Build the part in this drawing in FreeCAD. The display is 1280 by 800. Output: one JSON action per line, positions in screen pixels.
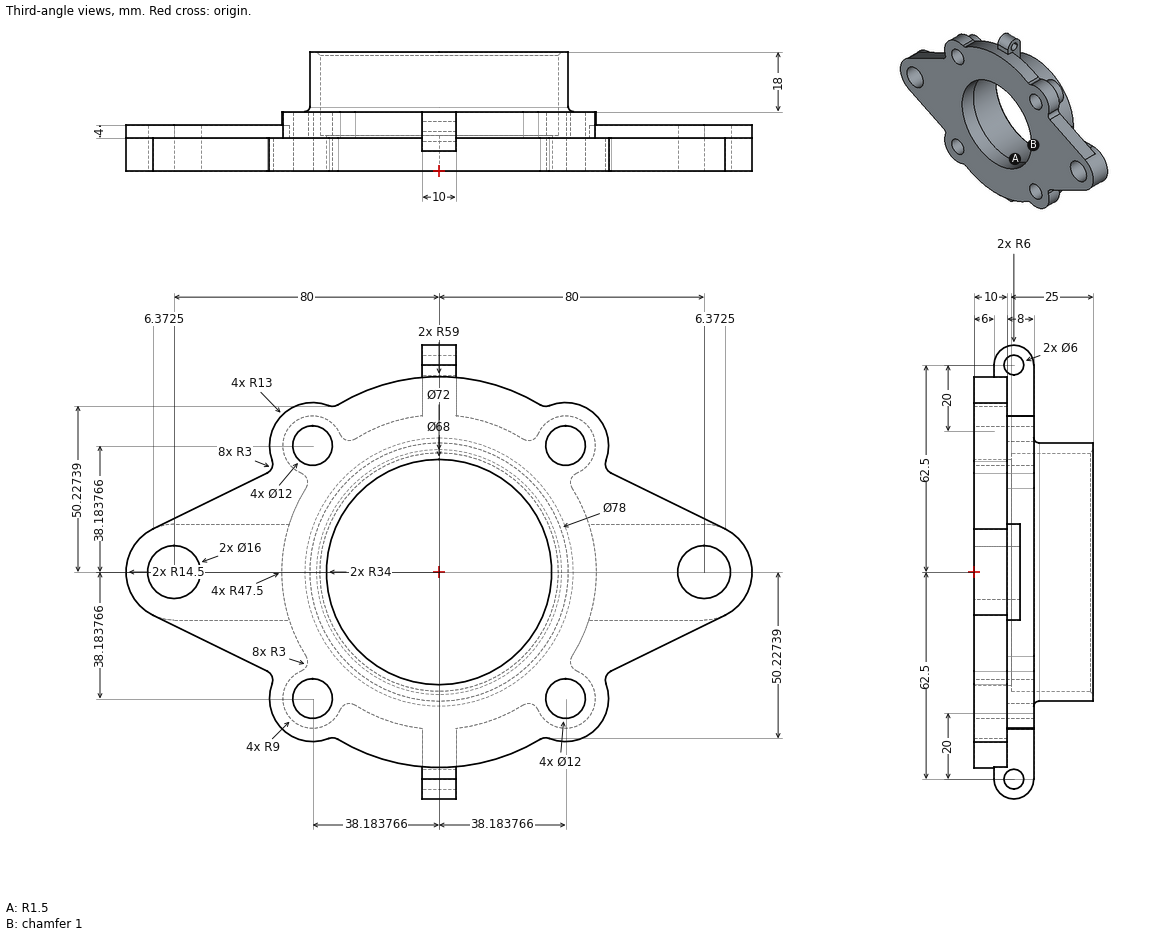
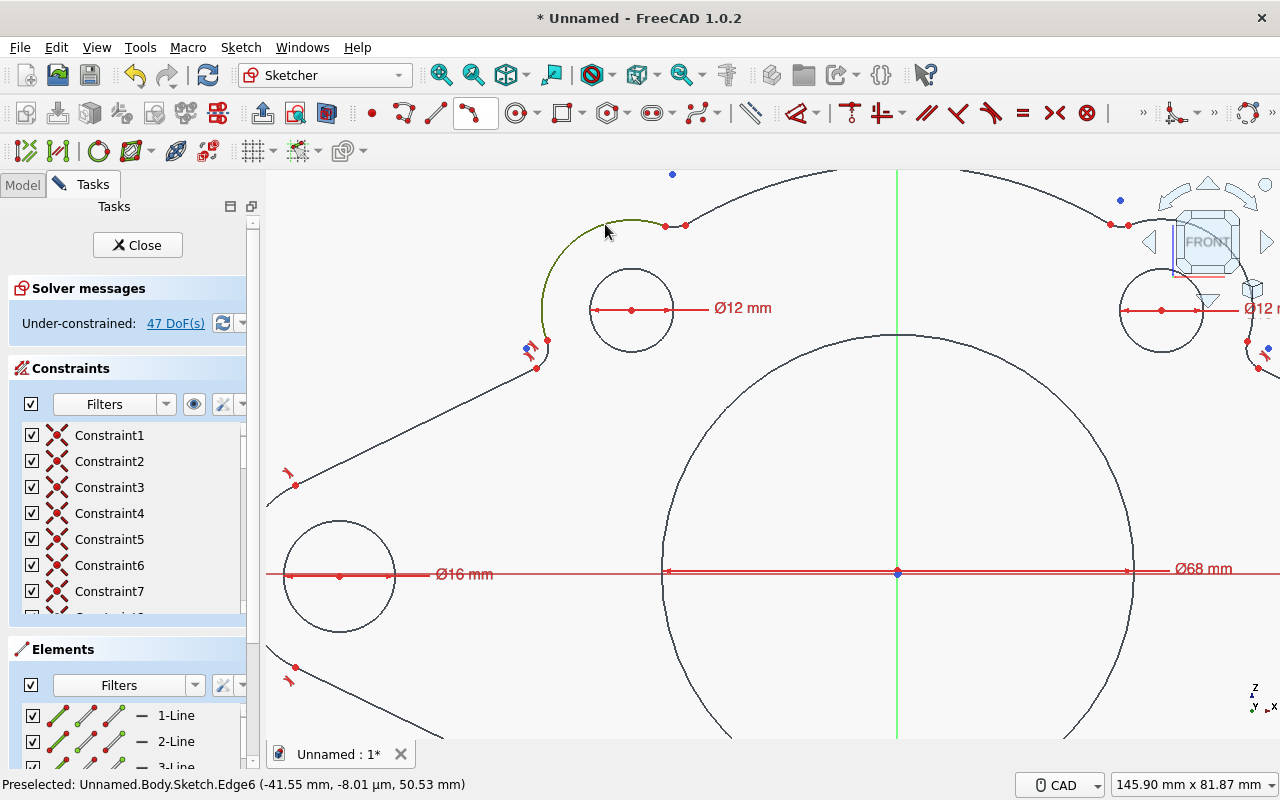
{"action": "scroll", "coordinate": [675, 227], "scroll_direction": "up", "scroll_amount": 2}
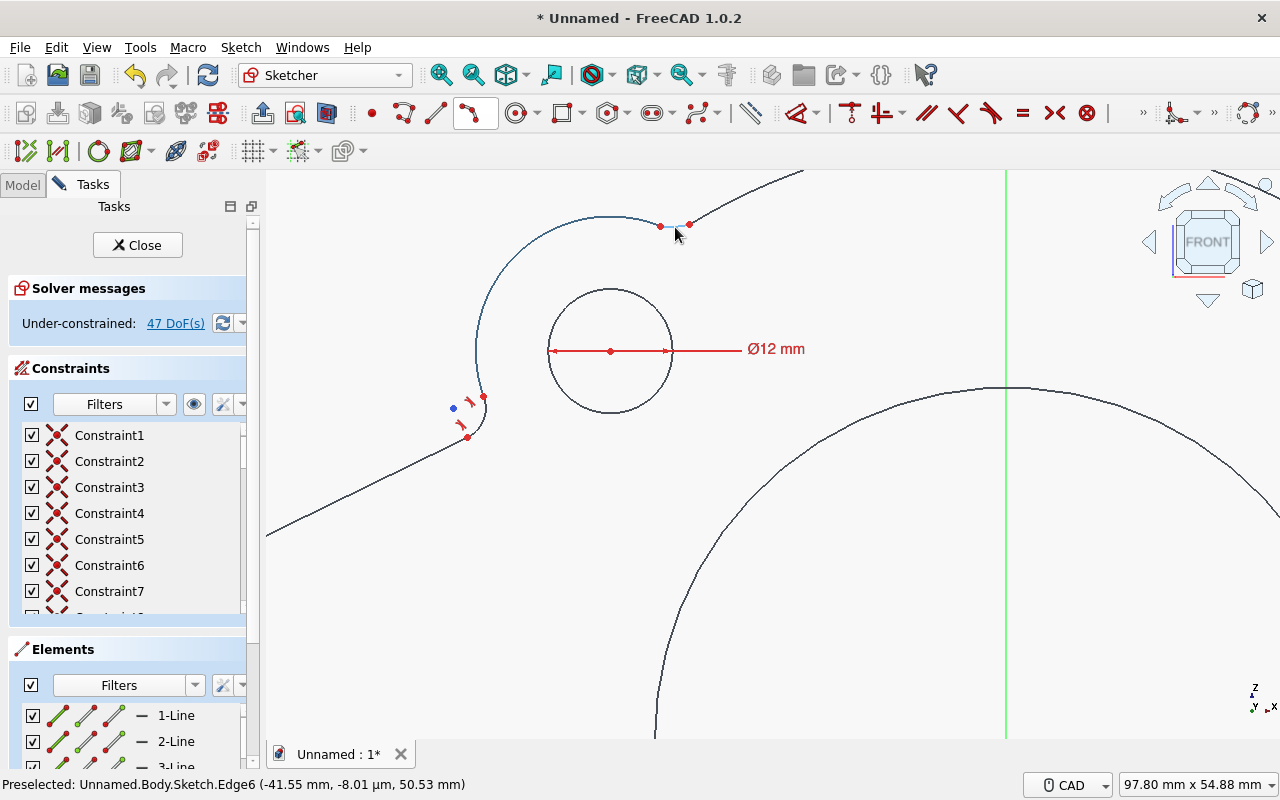
{"action": "left_click", "coordinate": [675, 227]}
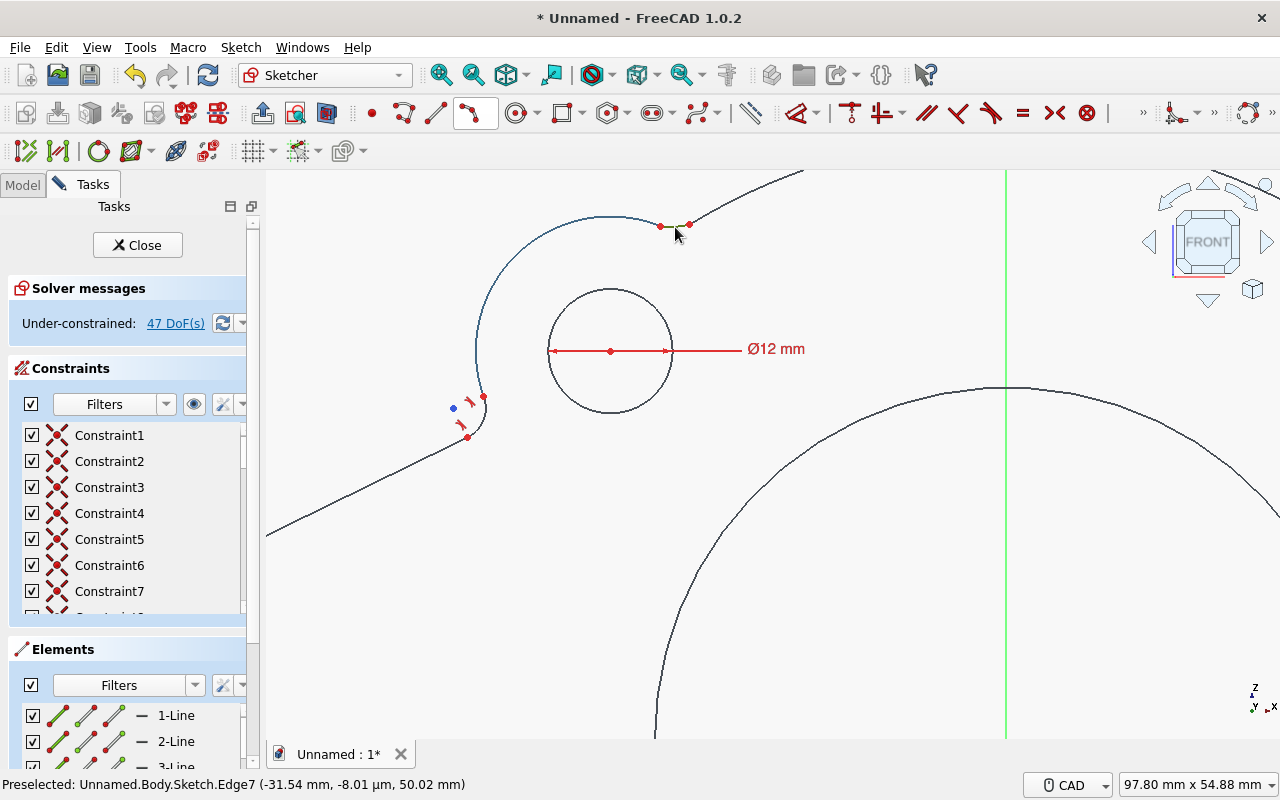
{"action": "left_click", "coordinate": [992, 114]}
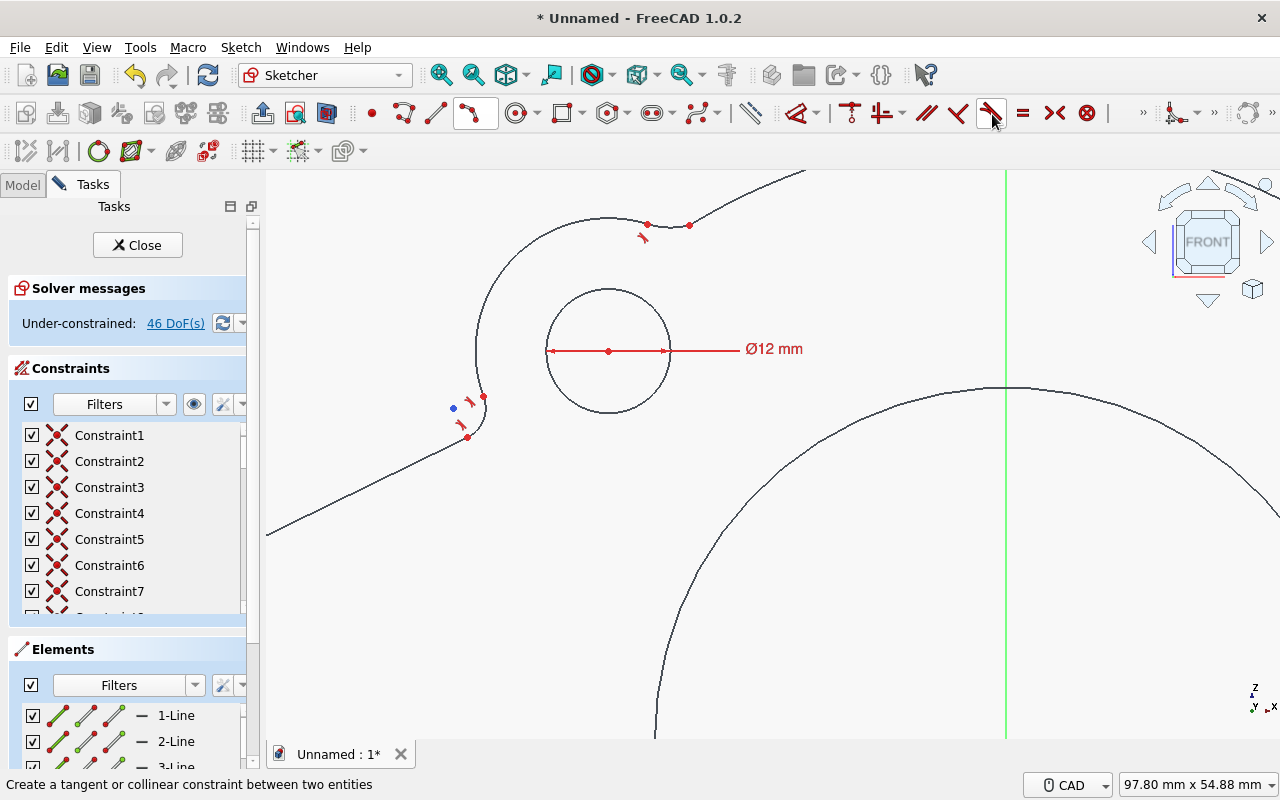
{"action": "left_click", "coordinate": [660, 227]}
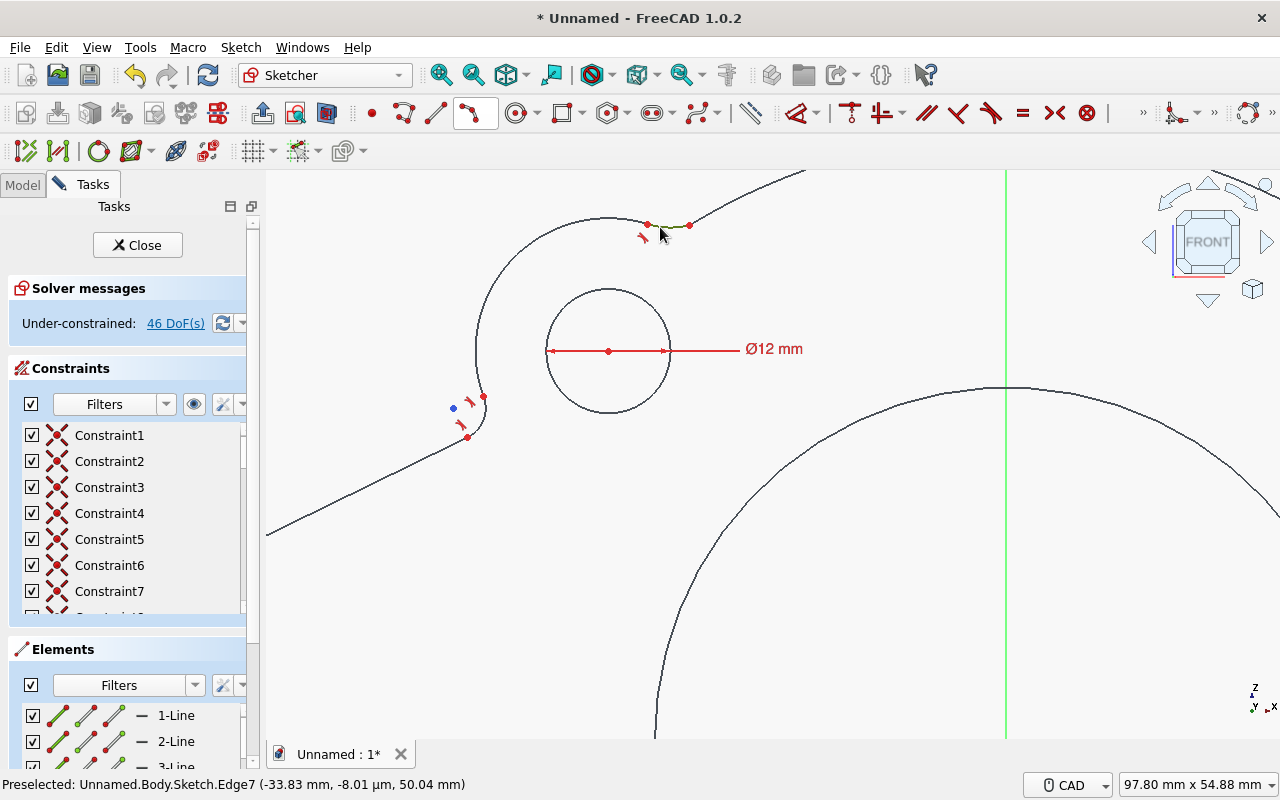
{"action": "scroll", "coordinate": [574, 329], "scroll_direction": "down", "scroll_amount": 6}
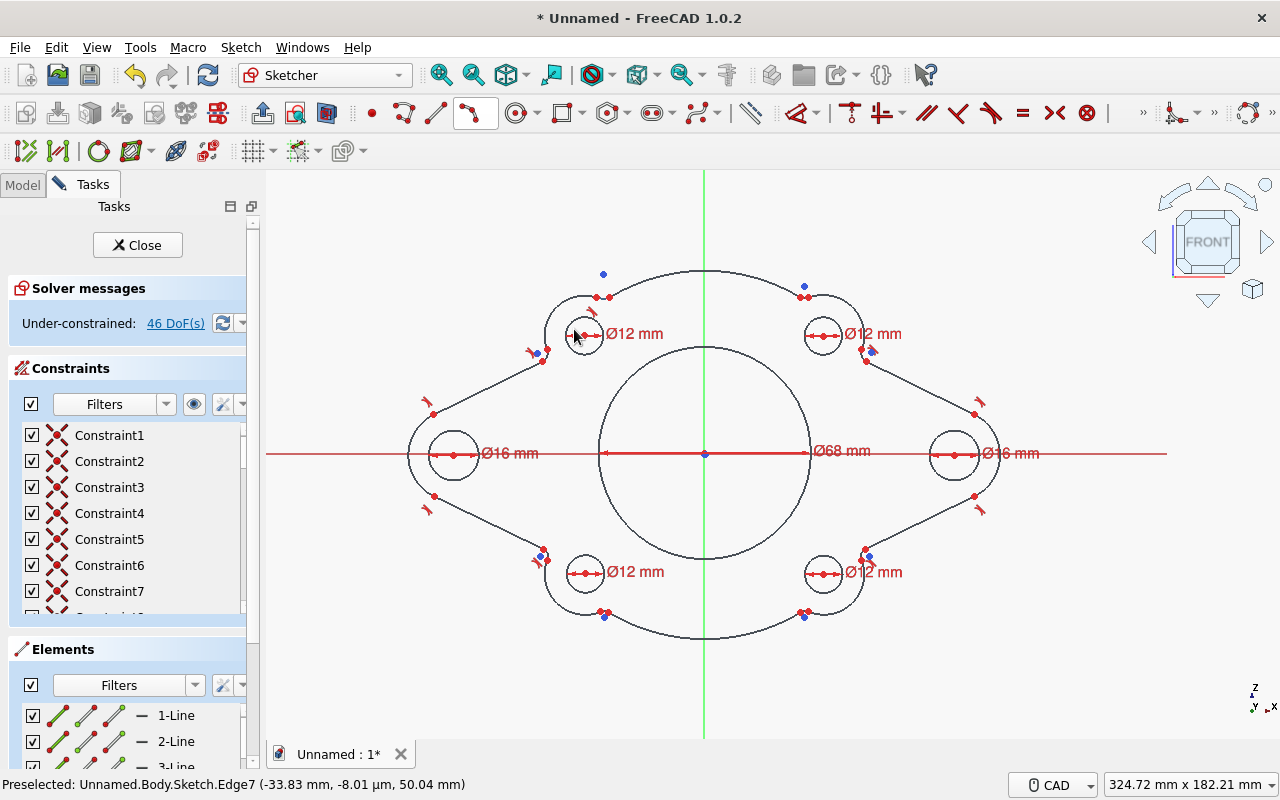
{"action": "left_click", "coordinate": [744, 275]}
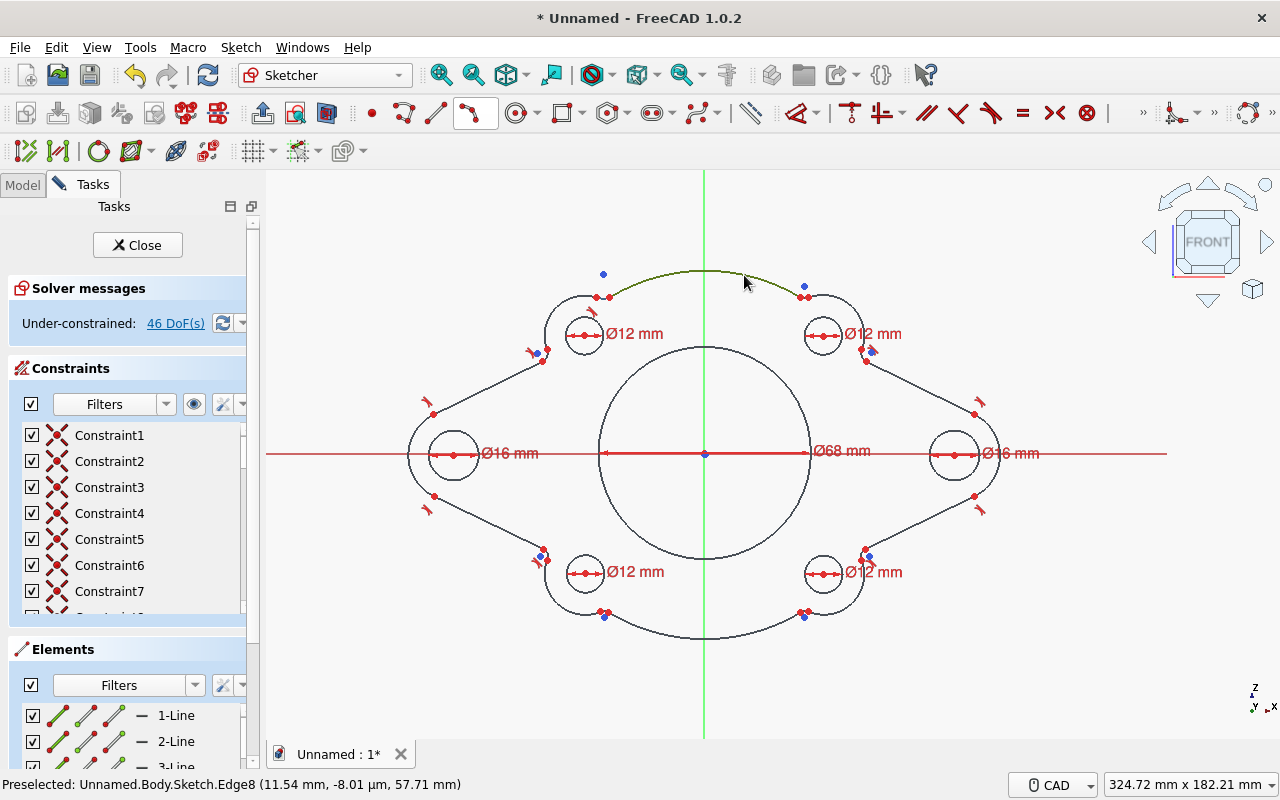
{"action": "left_click", "coordinate": [992, 114]}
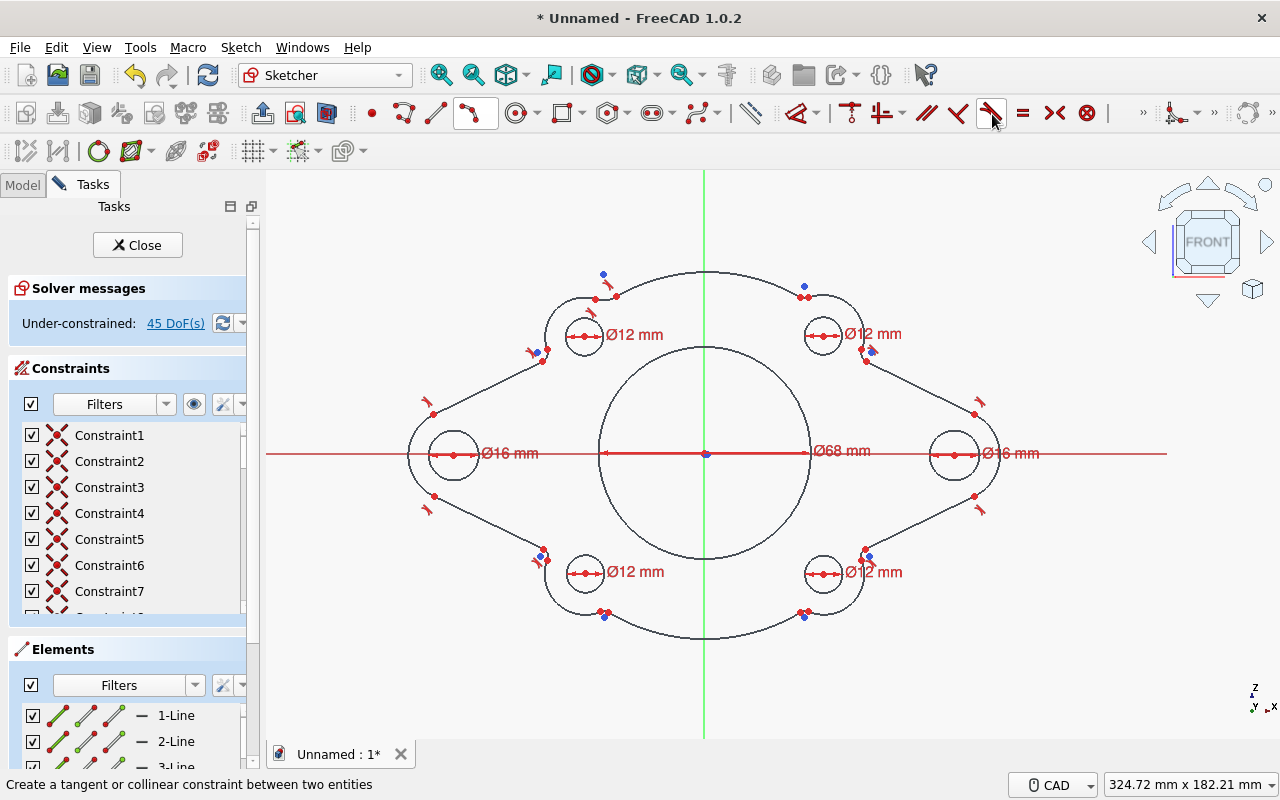
{"action": "left_click", "coordinate": [747, 276]}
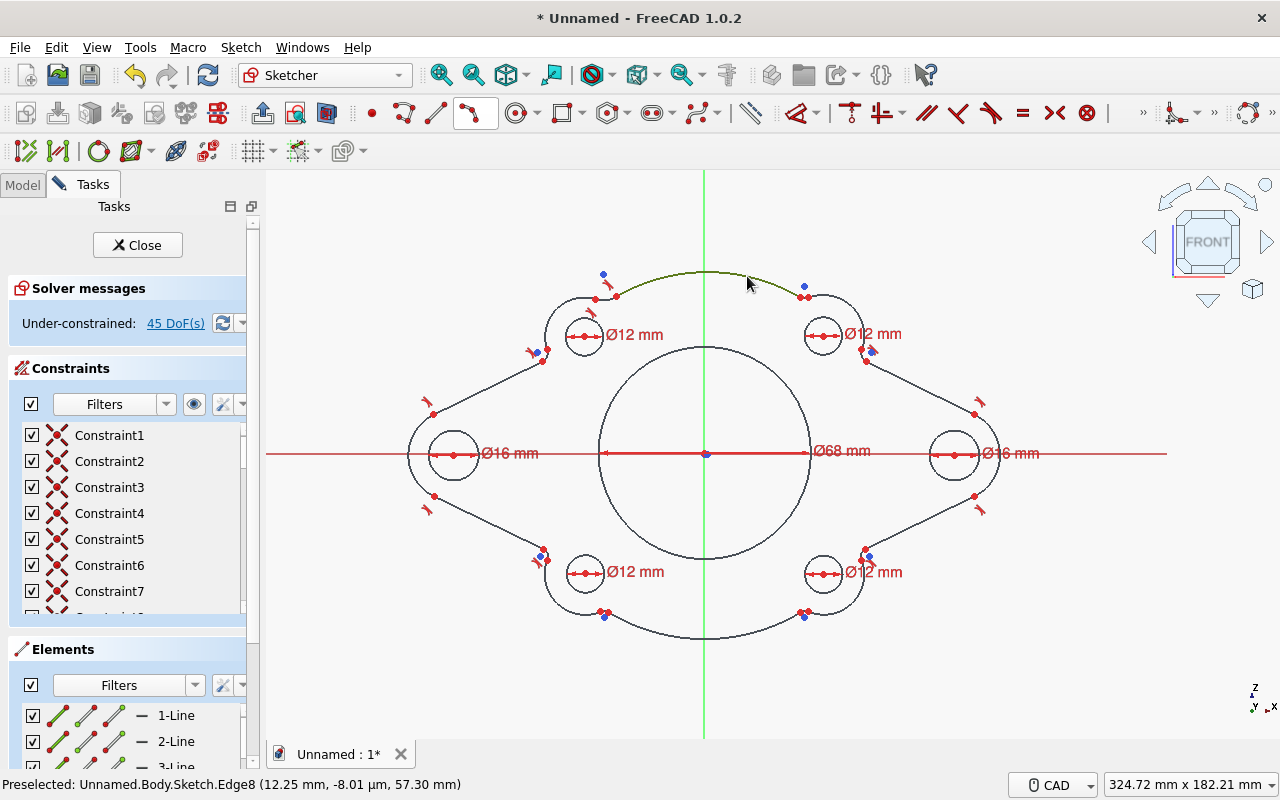
{"action": "scroll", "coordinate": [804, 298], "scroll_direction": "up", "scroll_amount": 7}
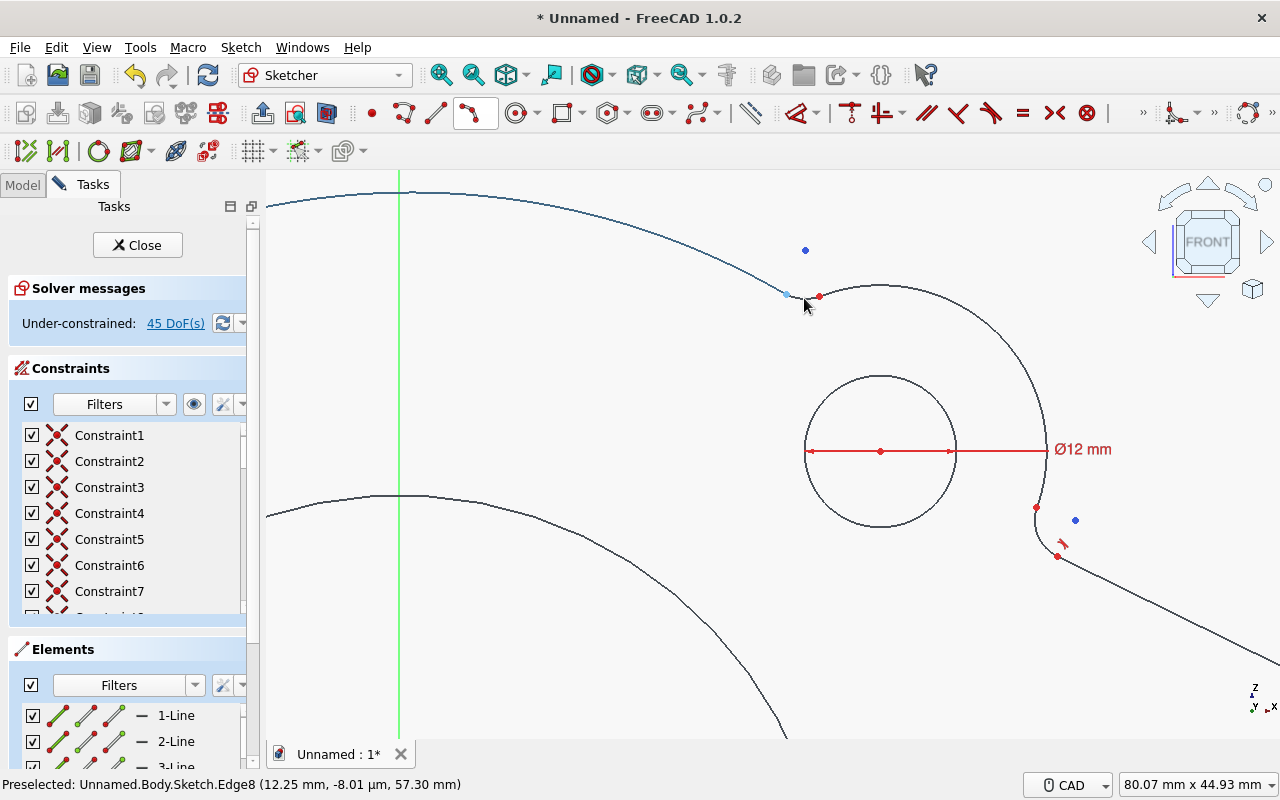
{"action": "left_click", "coordinate": [803, 299]}